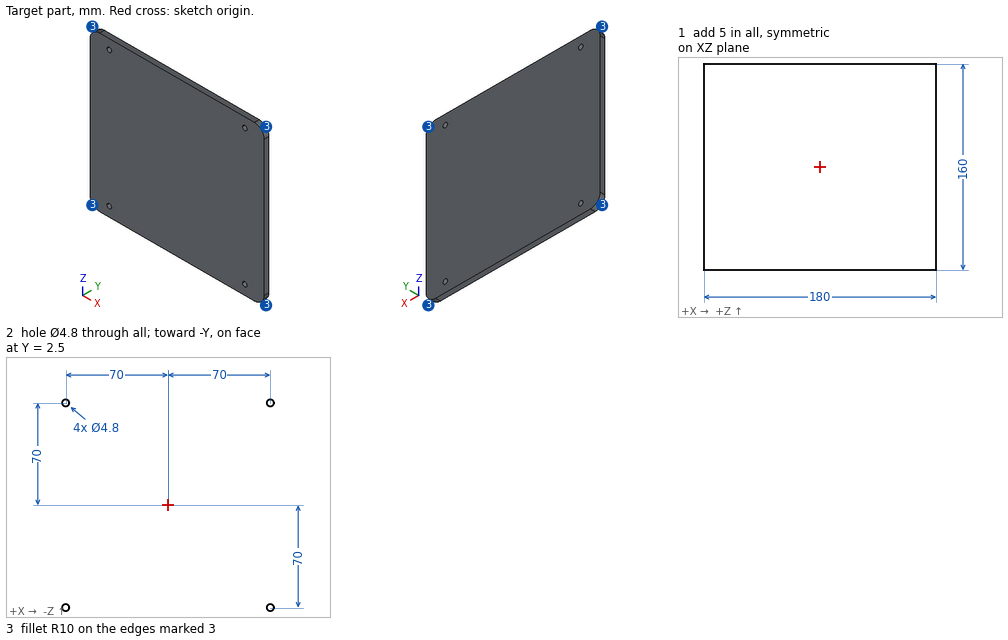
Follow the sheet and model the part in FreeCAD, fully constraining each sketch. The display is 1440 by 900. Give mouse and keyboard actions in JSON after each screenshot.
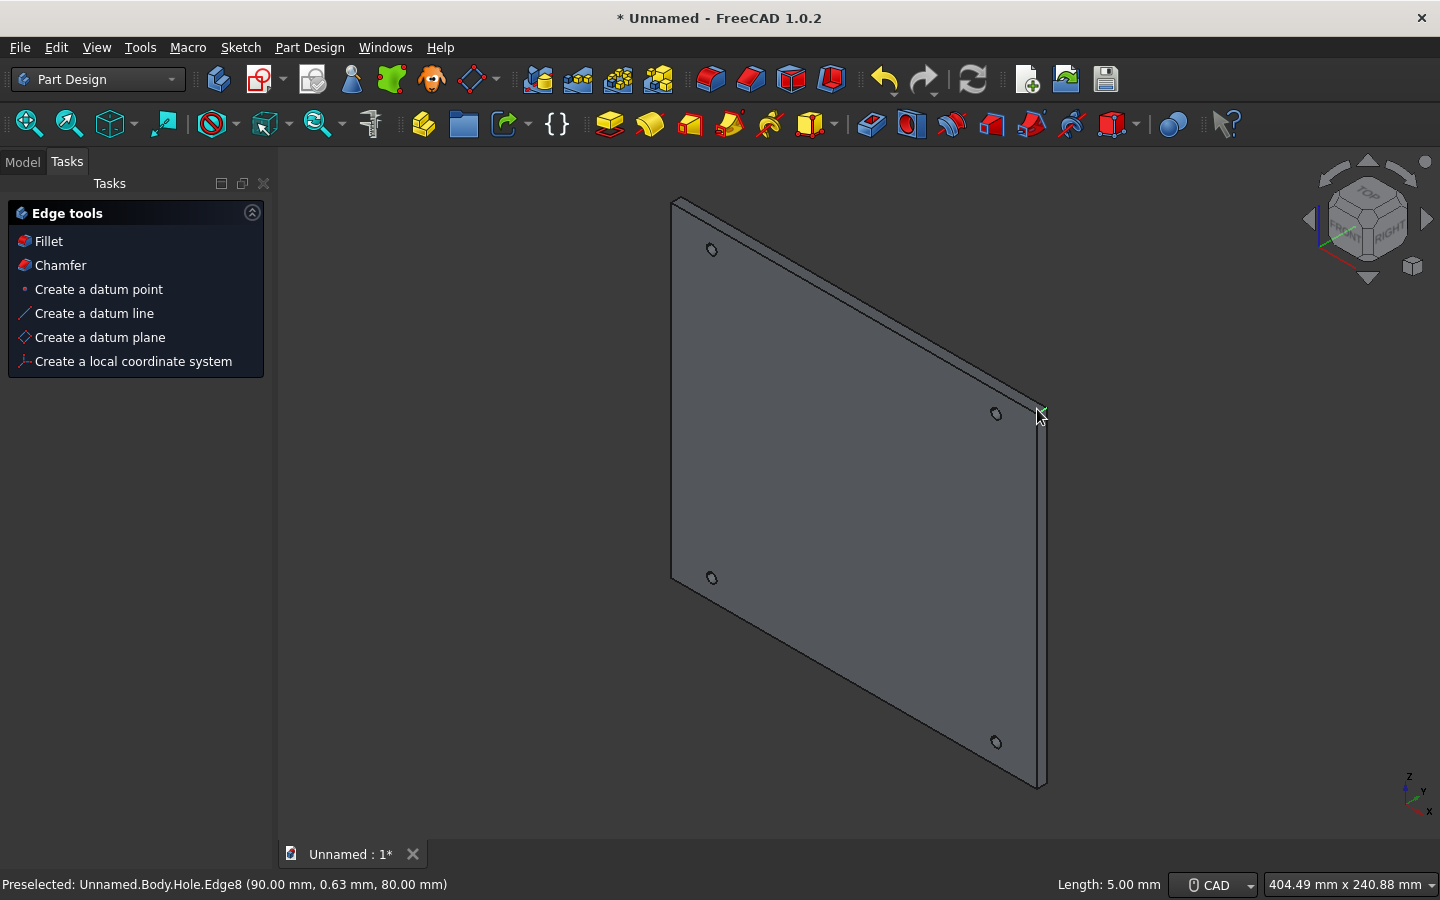
{"action": "scroll", "coordinate": [676, 199], "scroll_direction": "up", "scroll_amount": 6}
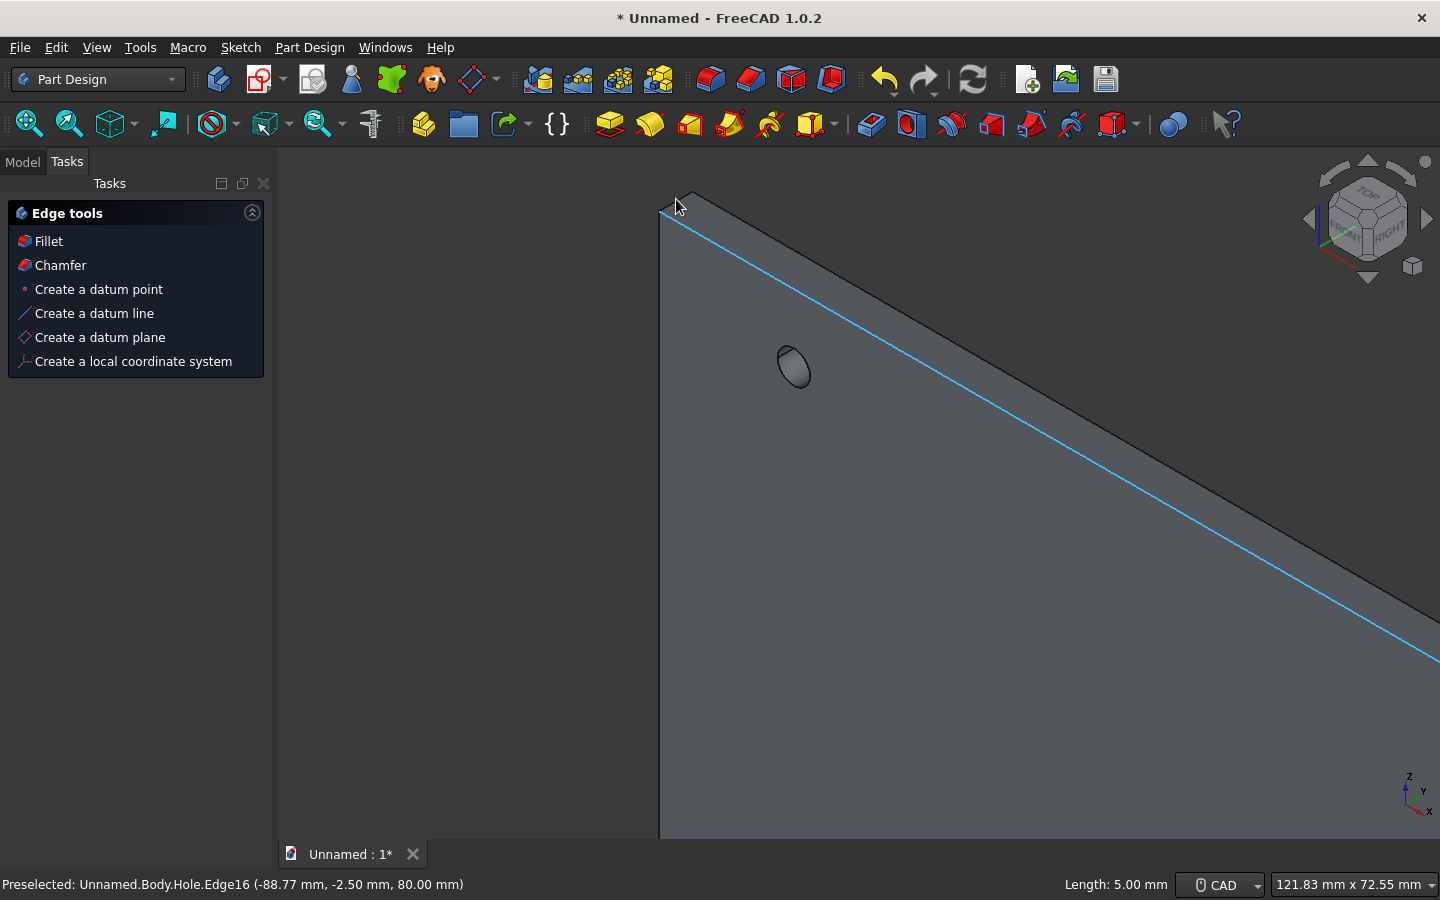
{"action": "left_click", "coordinate": [30, 124]}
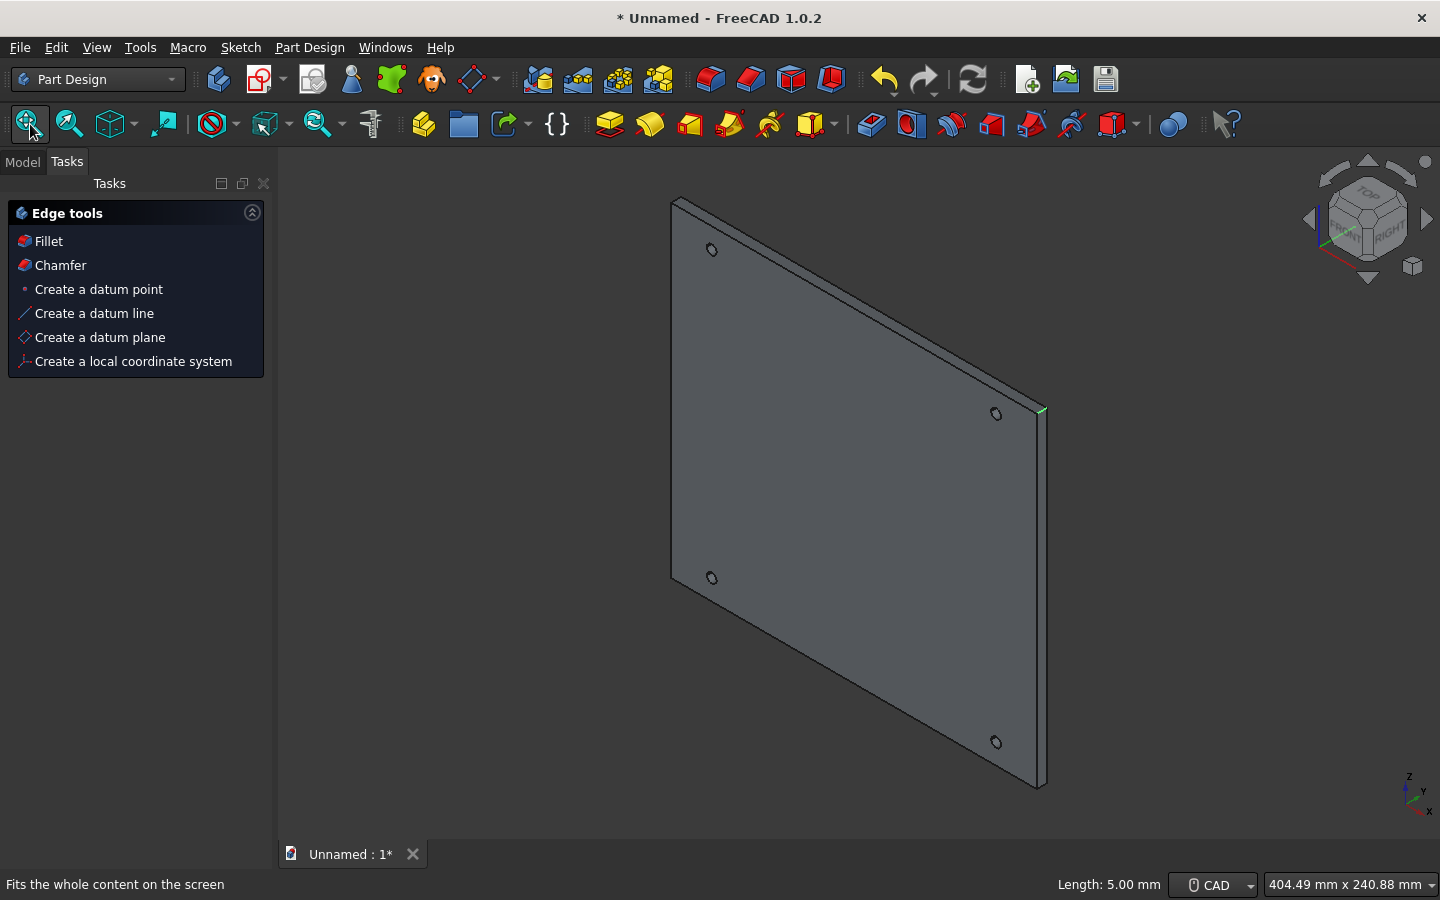
{"action": "key", "text": "2"}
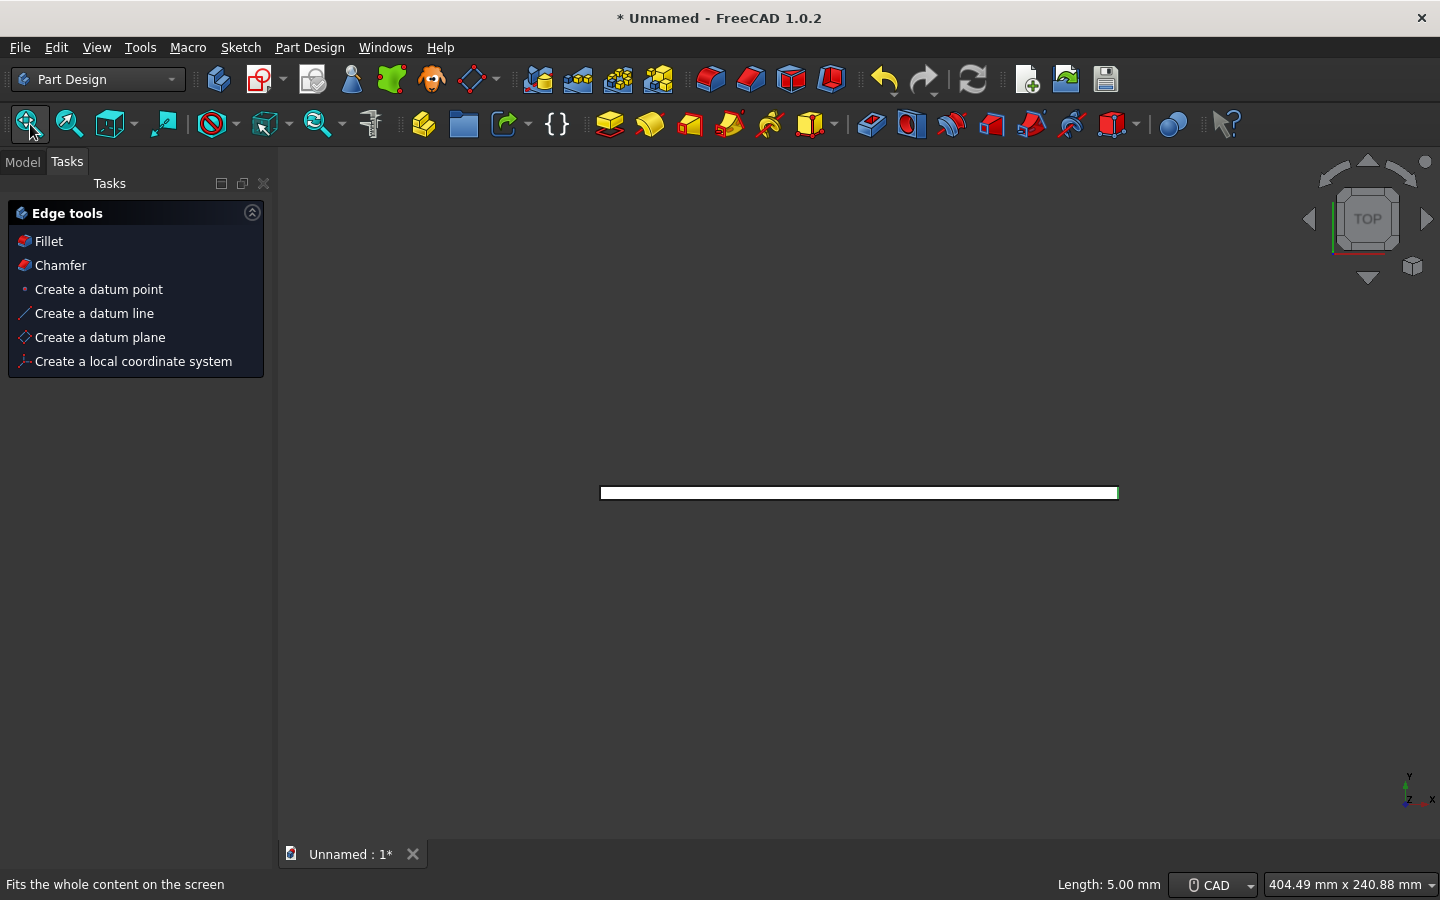
{"action": "key", "text": "v f"}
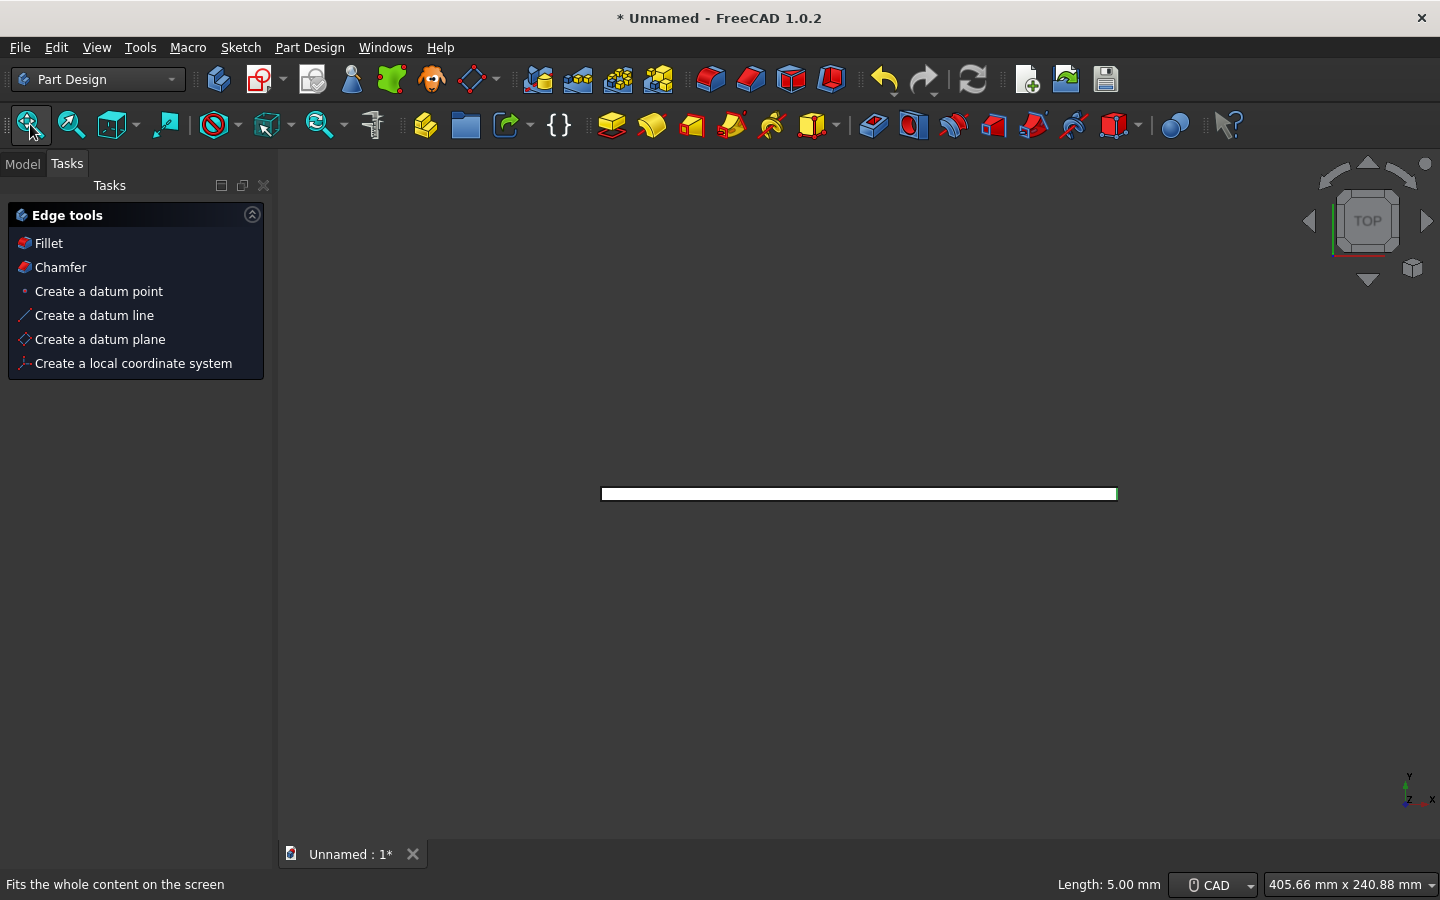
{"action": "left_click", "coordinate": [601, 493], "text": "ctrl"}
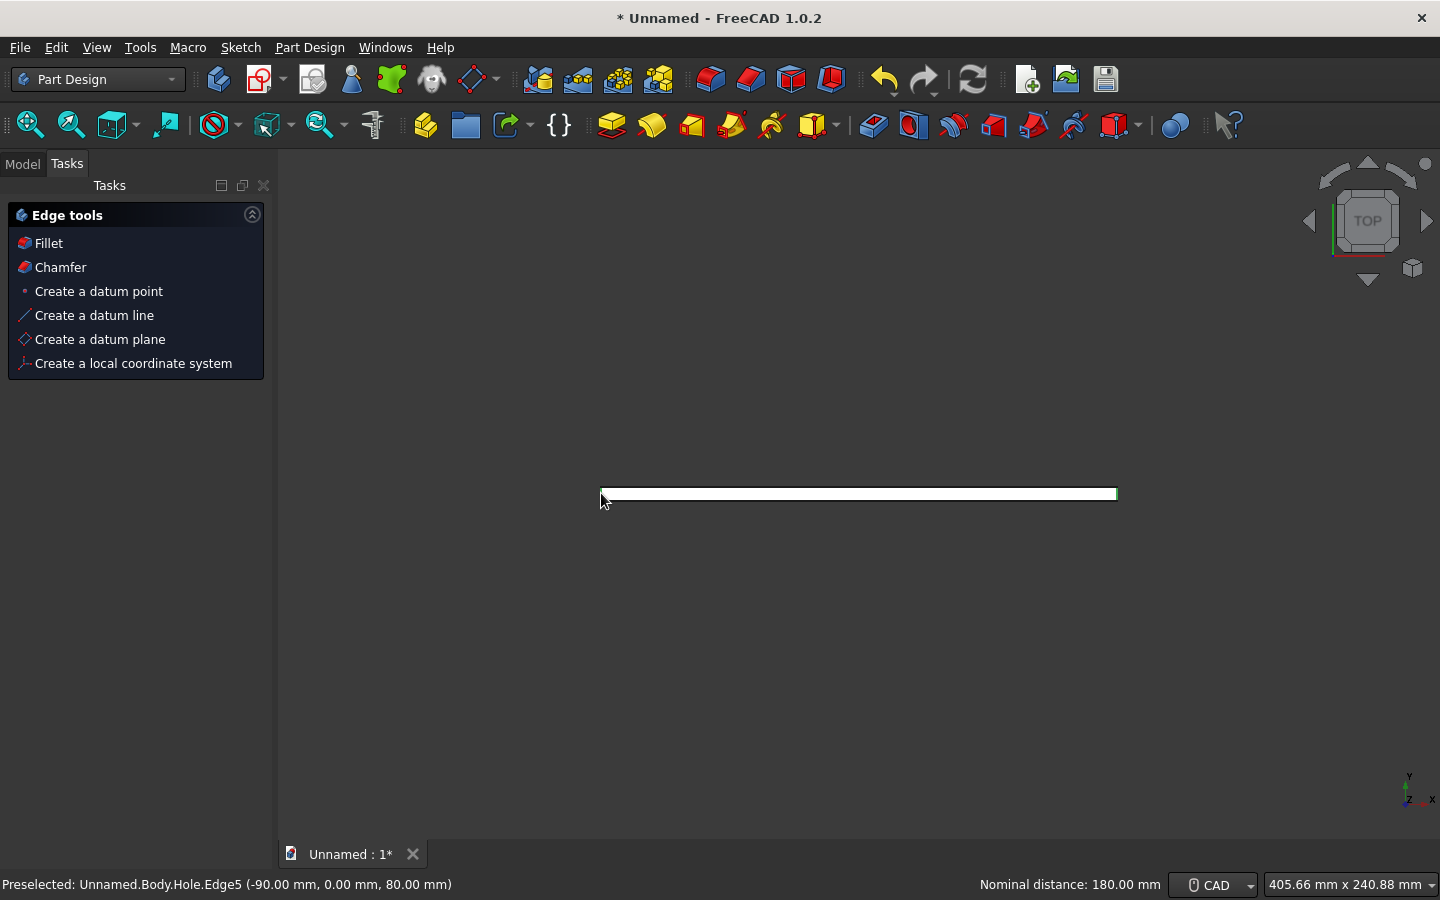
{"action": "scroll", "coordinate": [601, 493], "scroll_direction": "up", "scroll_amount": 6}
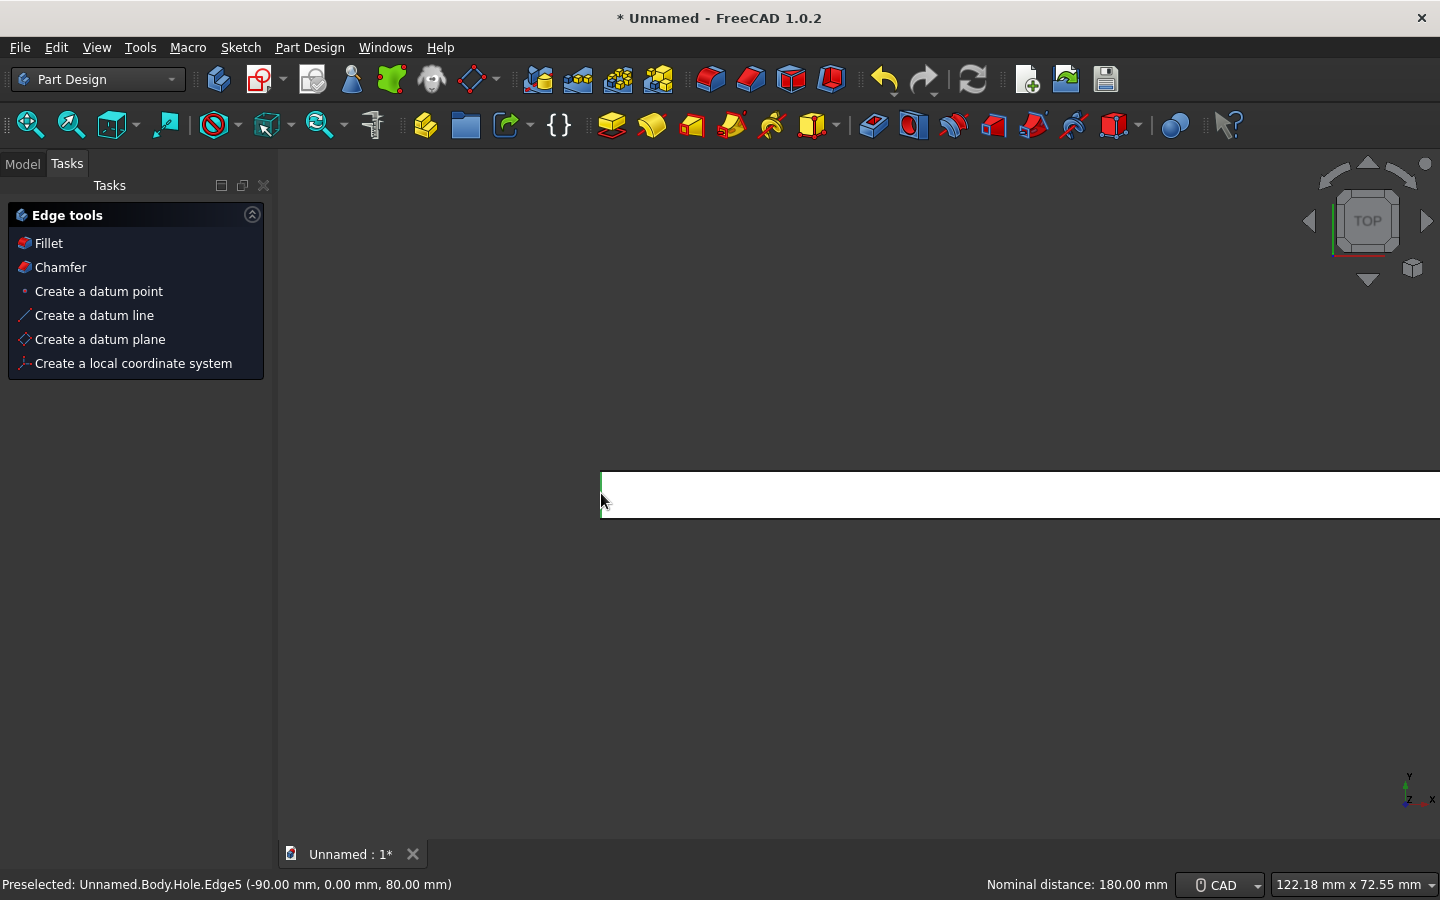
{"action": "key", "text": "v f"}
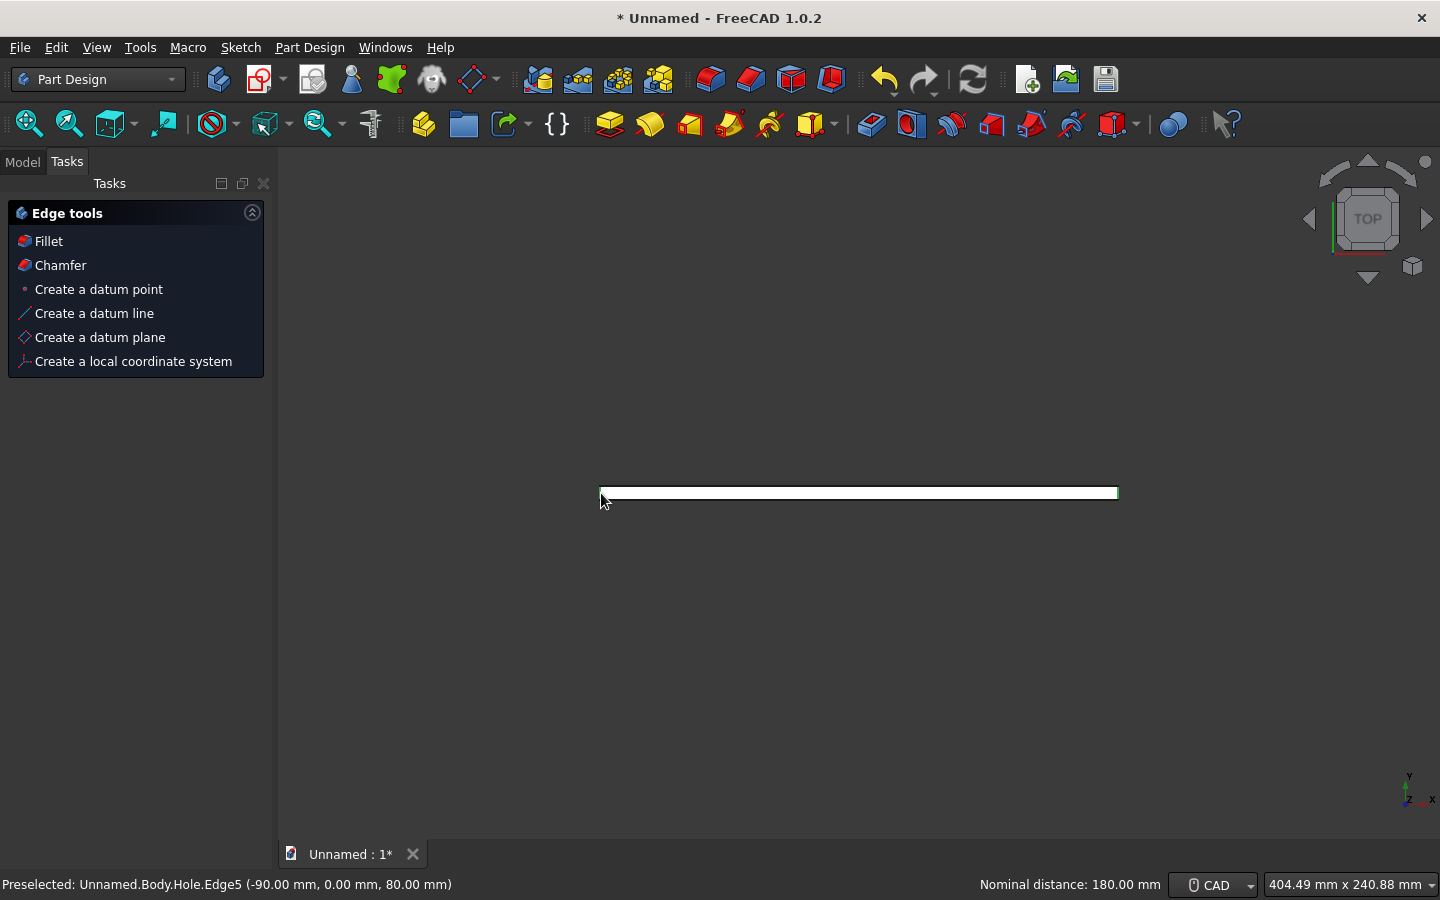
{"action": "key", "text": "1"}